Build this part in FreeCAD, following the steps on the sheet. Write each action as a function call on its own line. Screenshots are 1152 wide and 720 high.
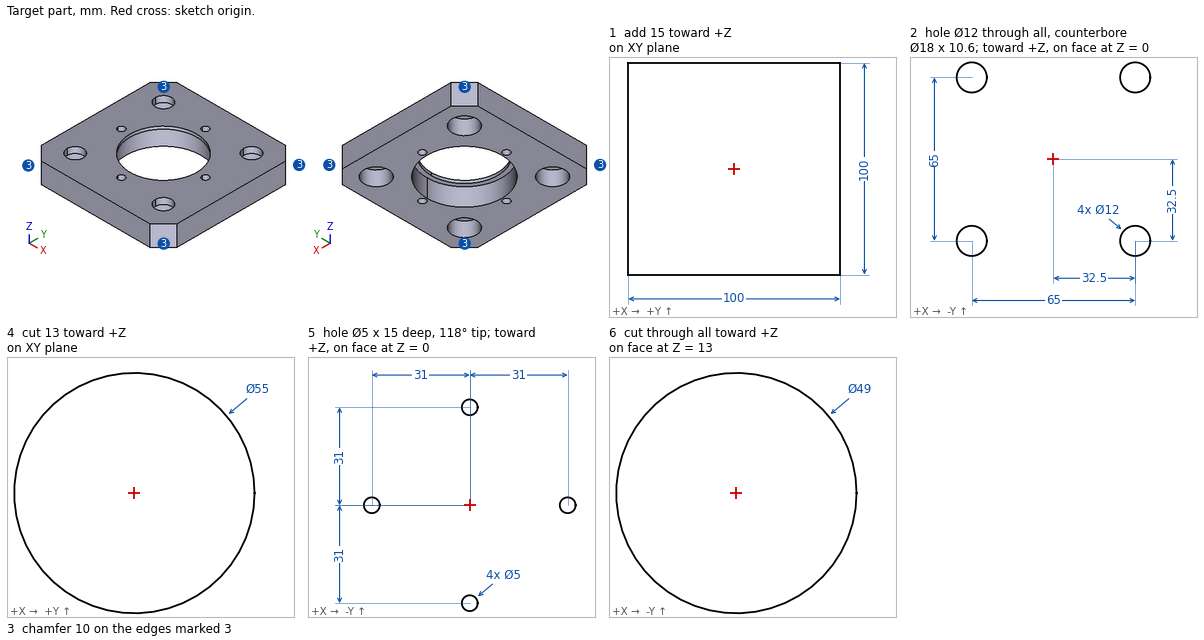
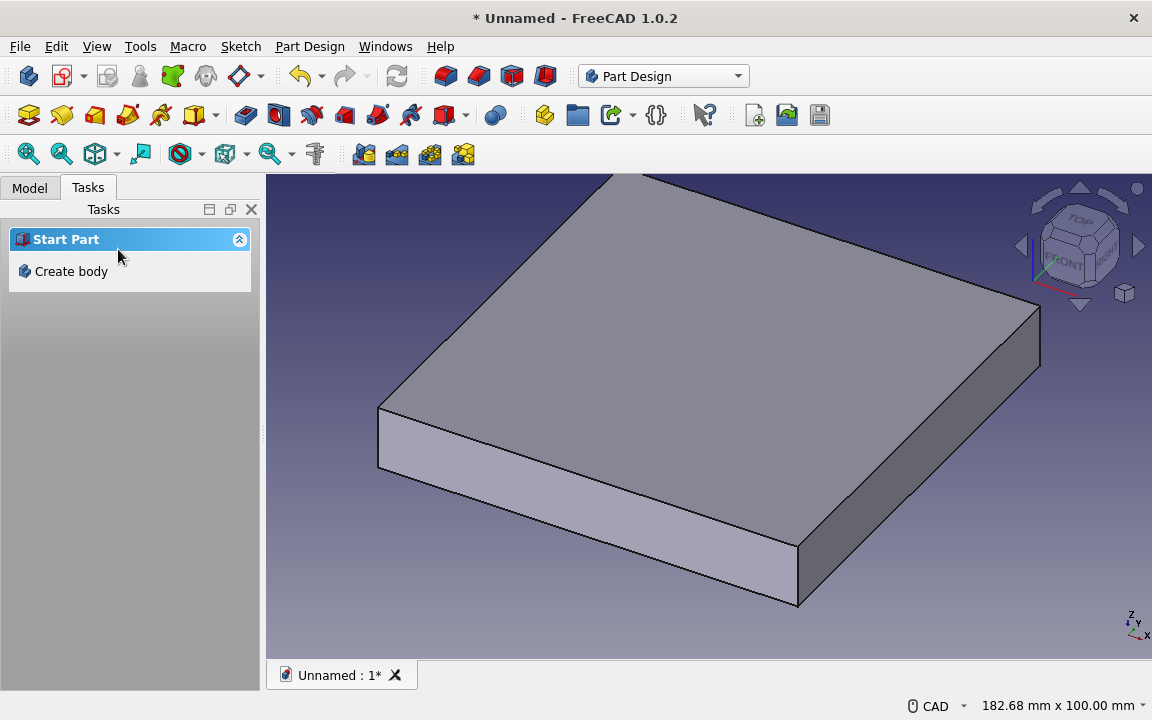
click(29, 154)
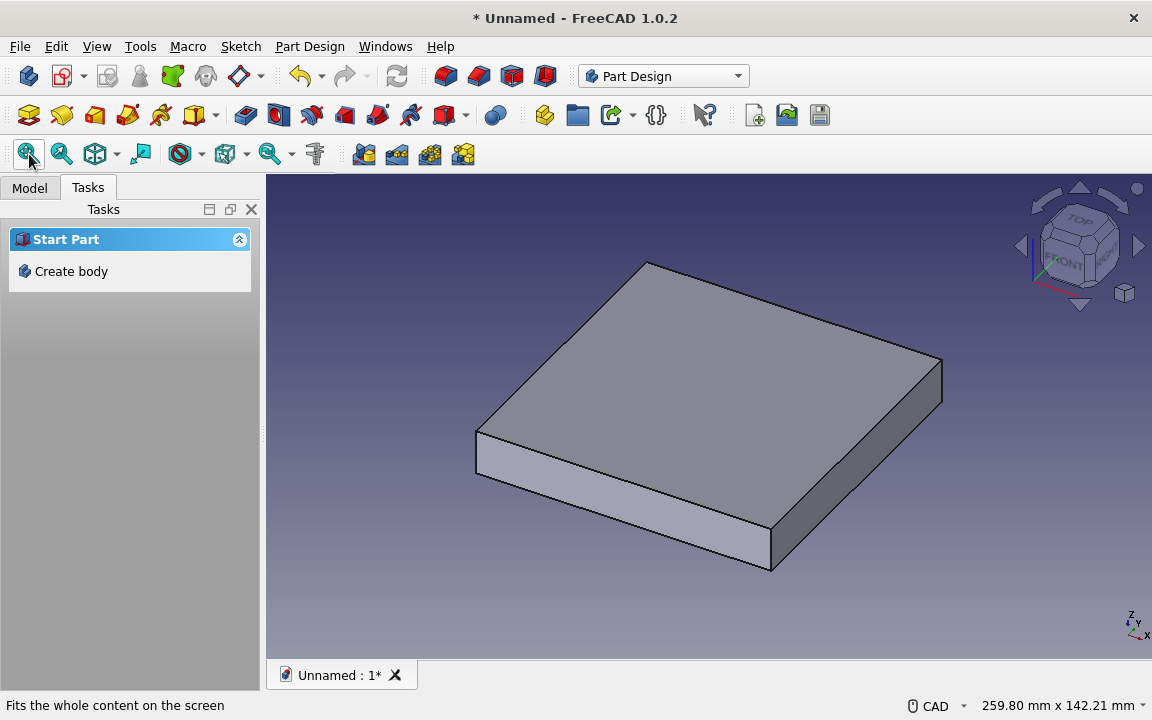
key(5)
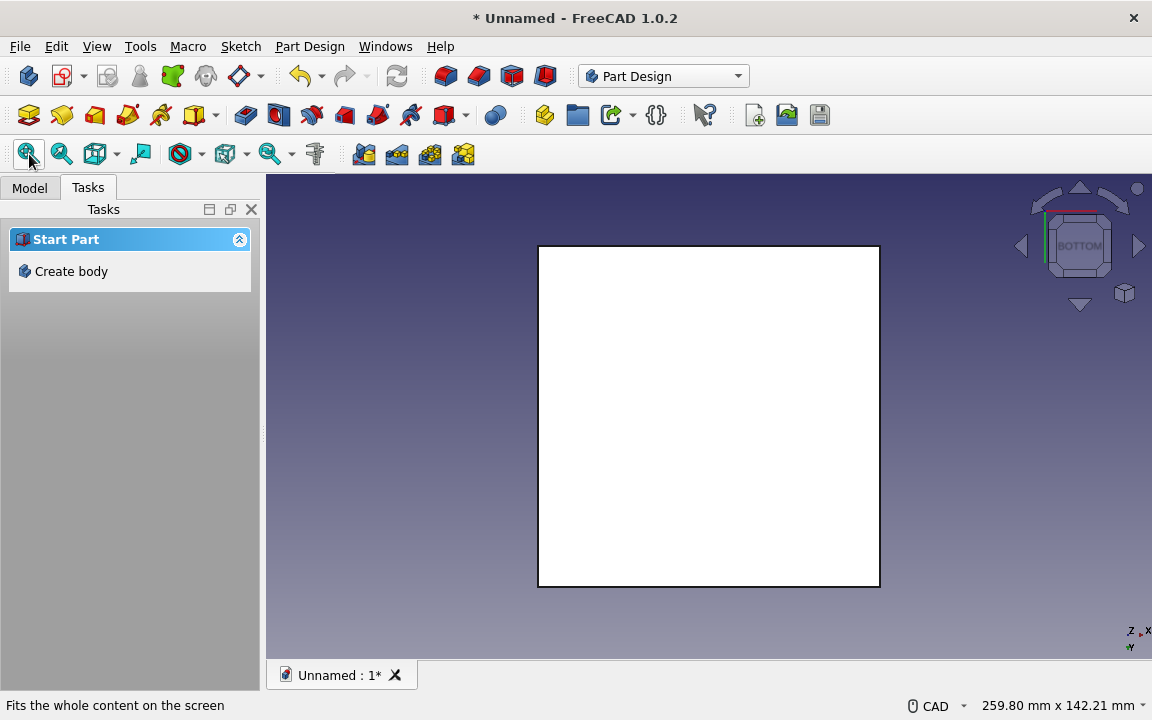
click(709, 415)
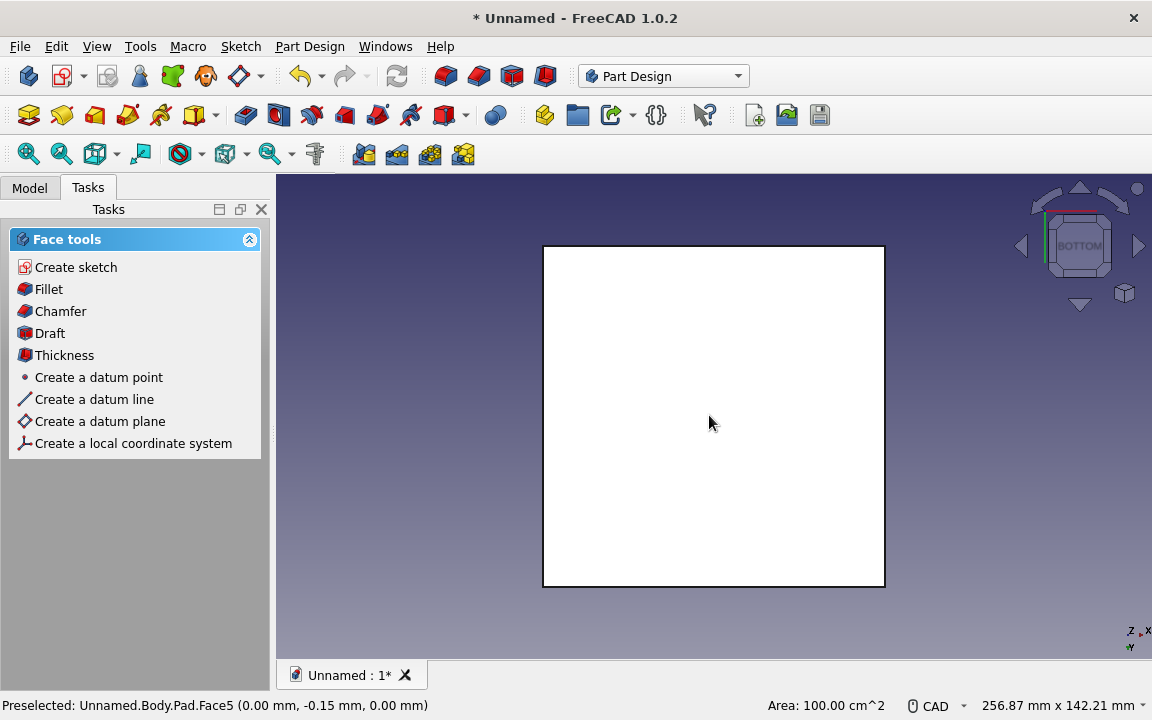
click(62, 76)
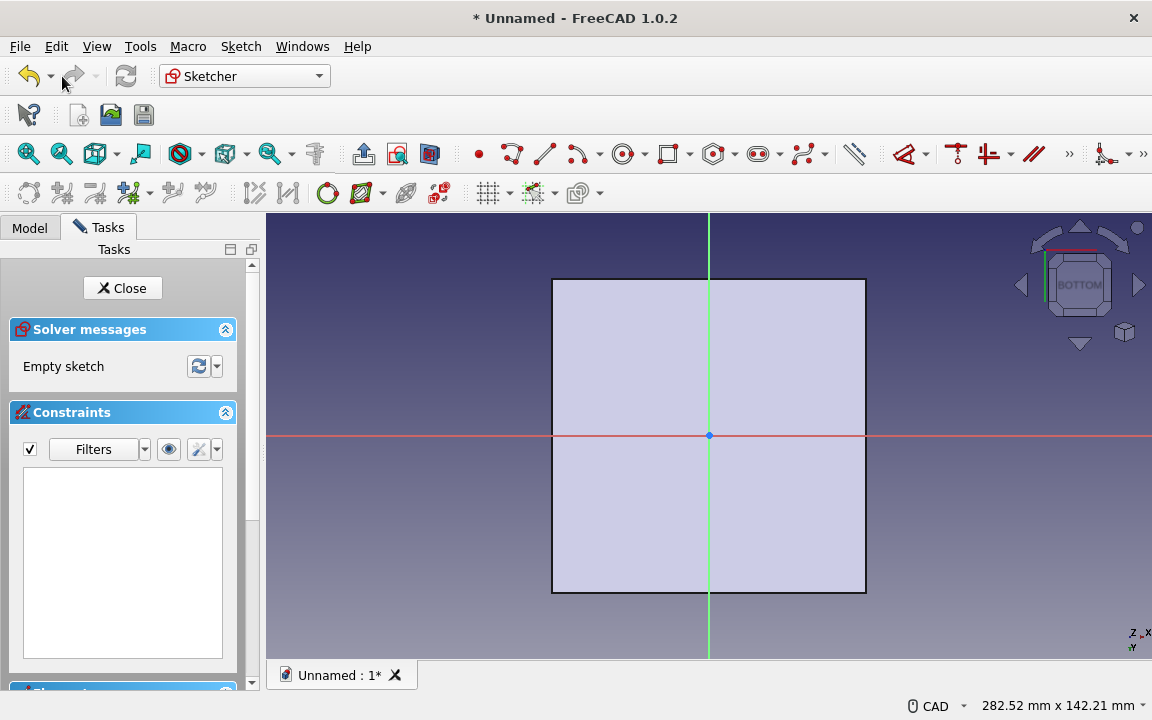
click(622, 154)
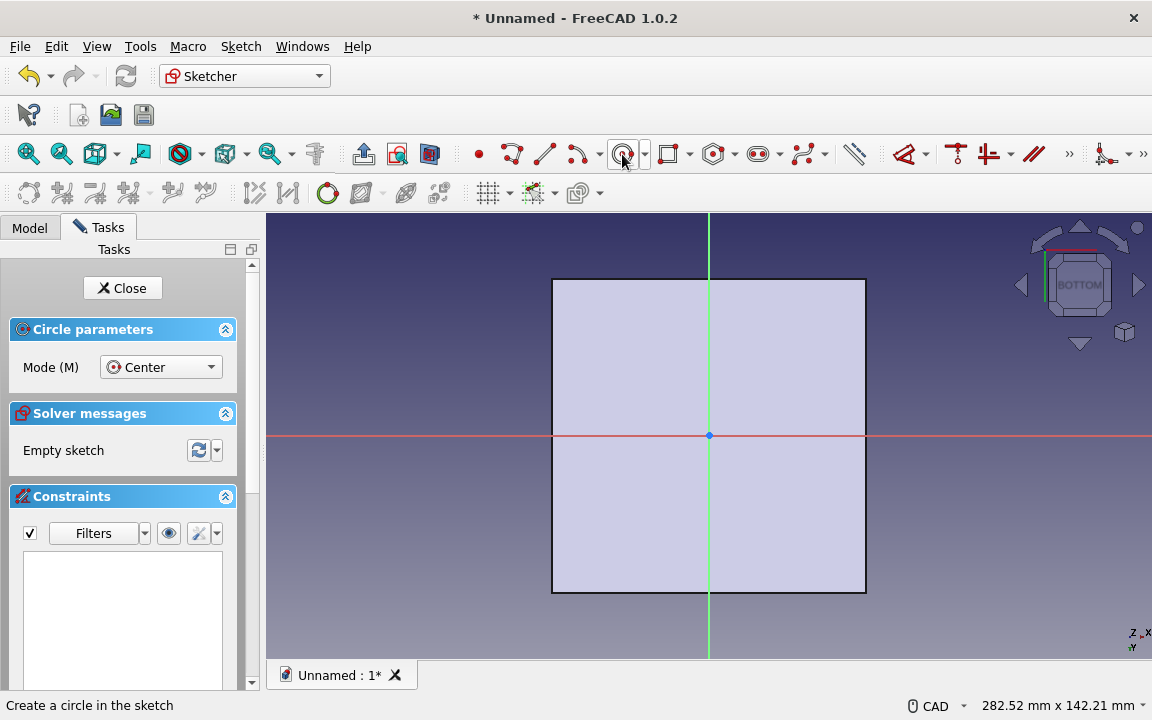
click(811, 538)
move(824, 525)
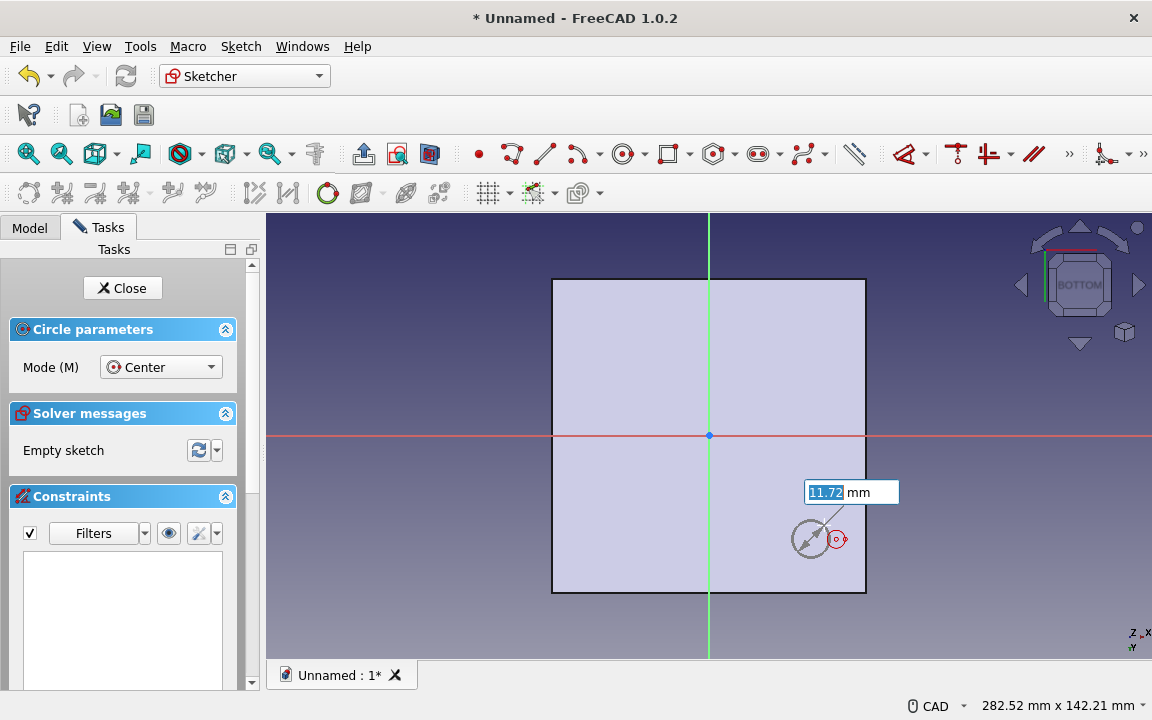
text(12)
key(Return)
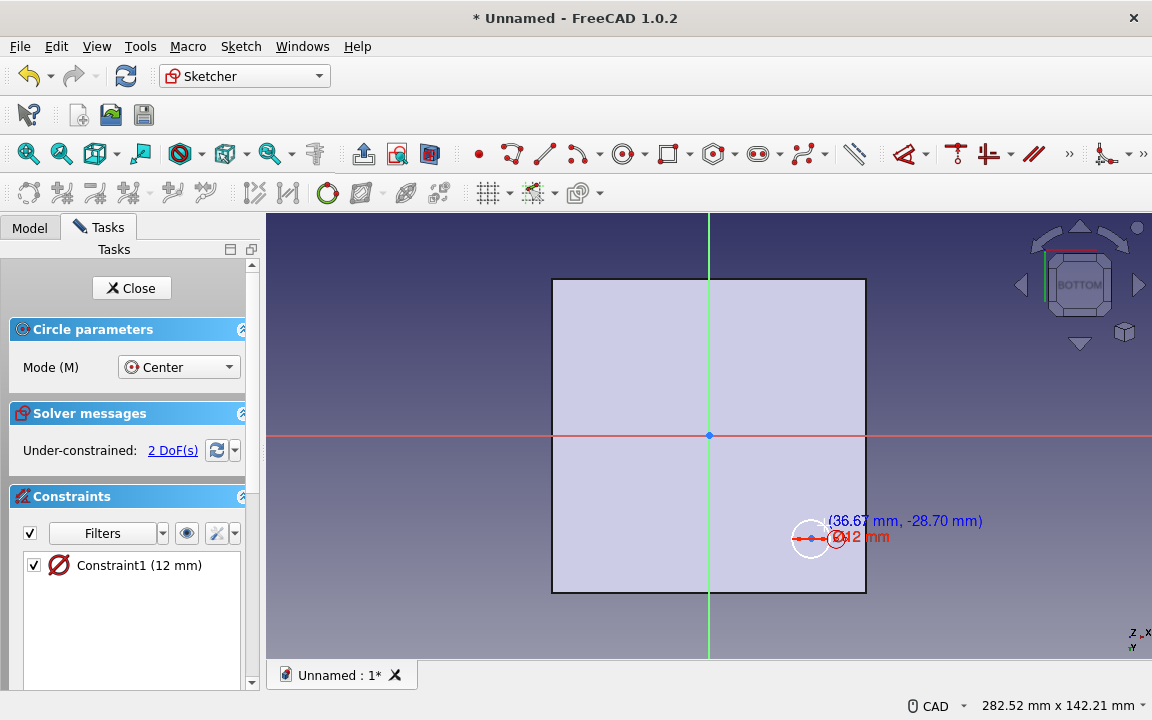
click(607, 538)
move(620, 525)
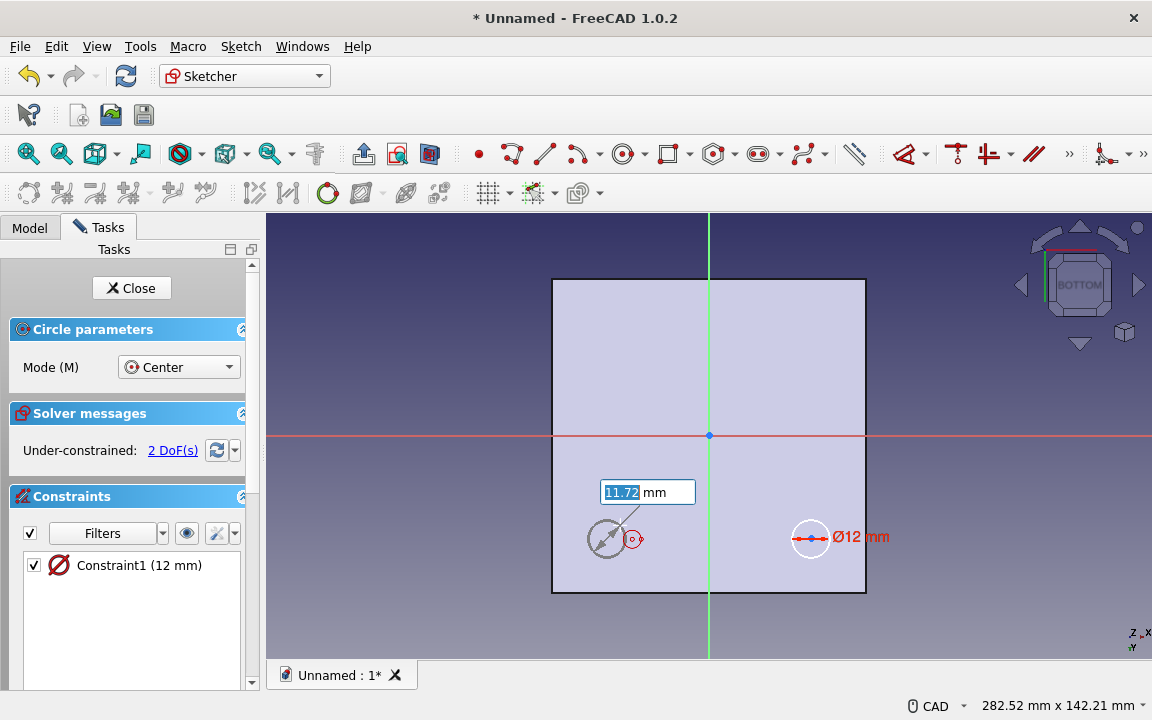
text(12)
key(Return)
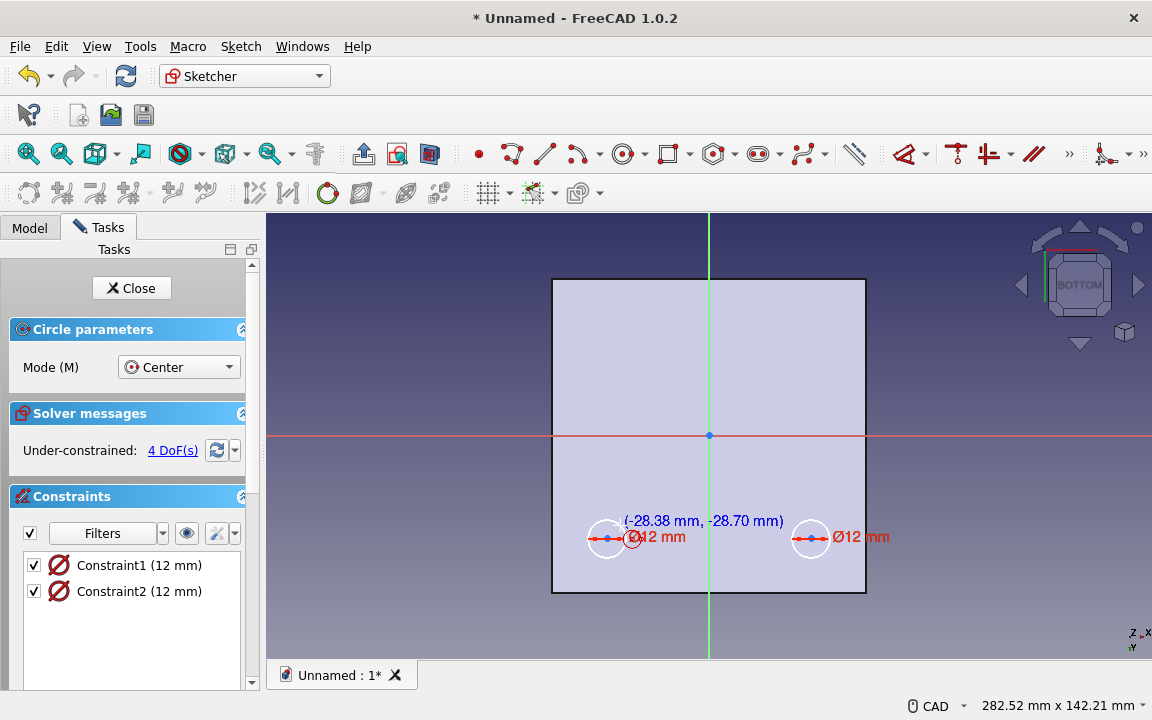
click(607, 334)
move(620, 321)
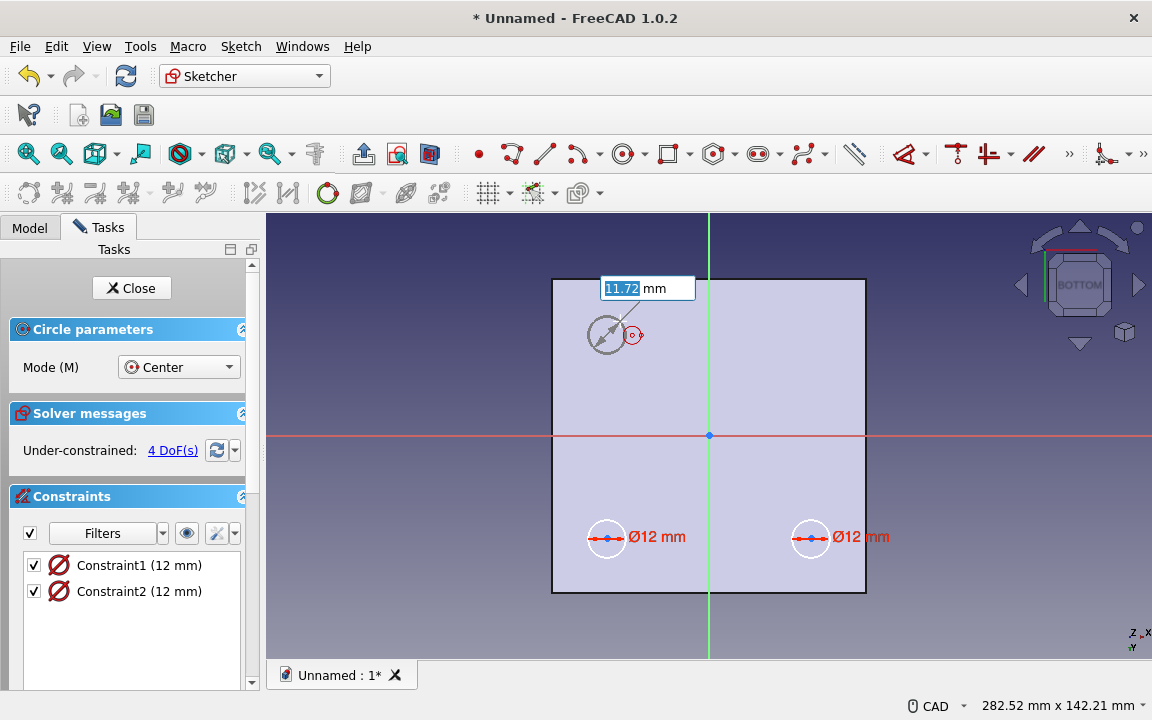
text(12)
key(Return)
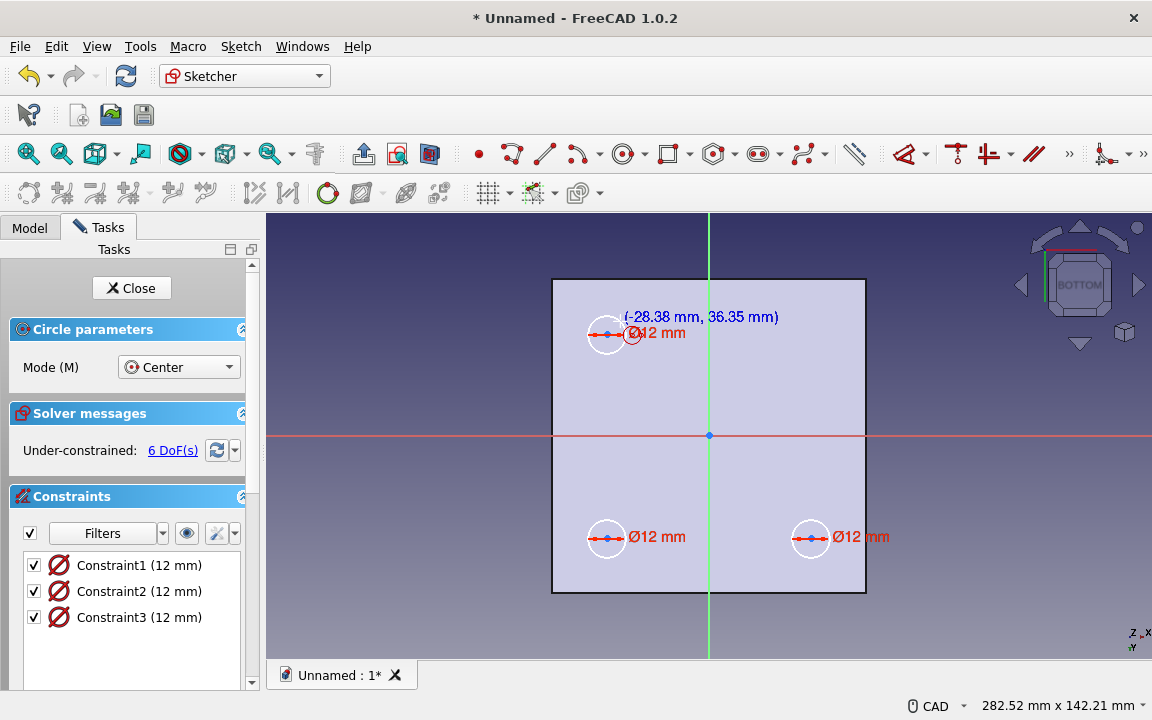
click(811, 334)
move(824, 321)